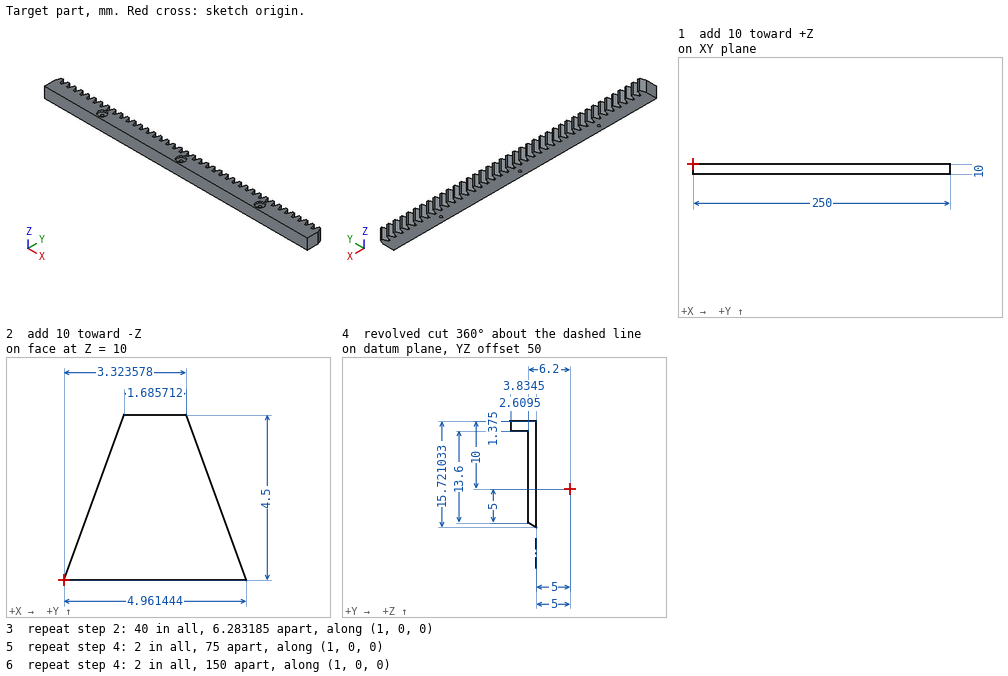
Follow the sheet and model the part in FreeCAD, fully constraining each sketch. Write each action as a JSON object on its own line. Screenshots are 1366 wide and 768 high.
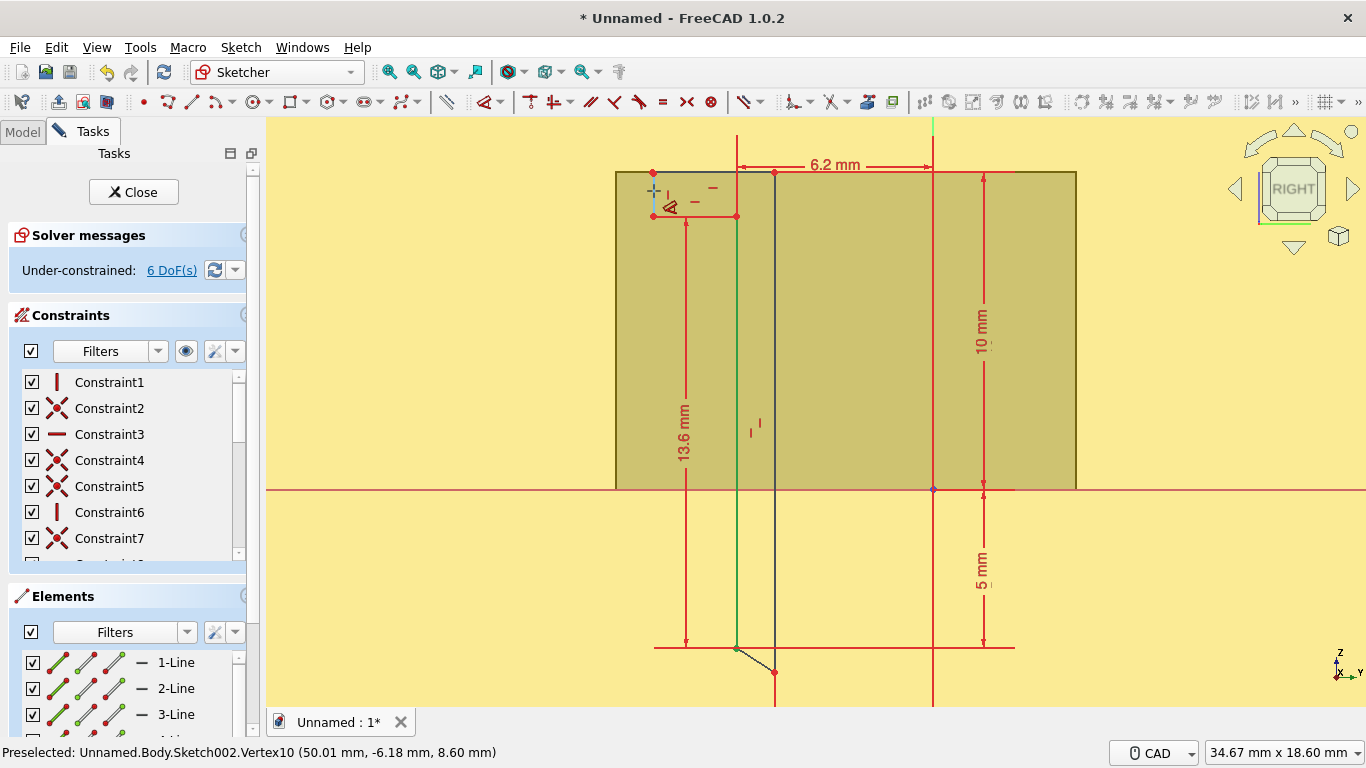
{"action": "left_click", "coordinate": [654, 191]}
{"action": "left_click", "coordinate": [620, 195]}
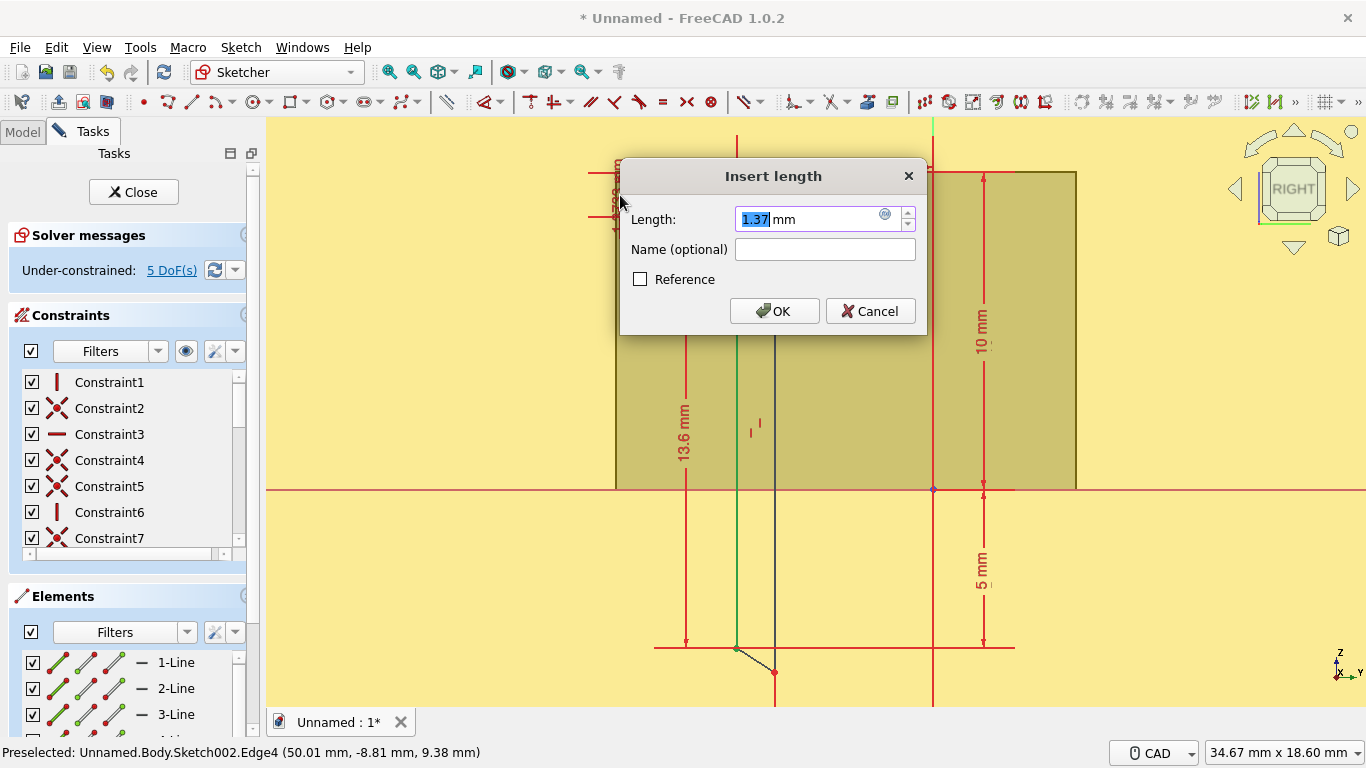
{"action": "type", "text": "1.375"}
{"action": "key", "text": "Return"}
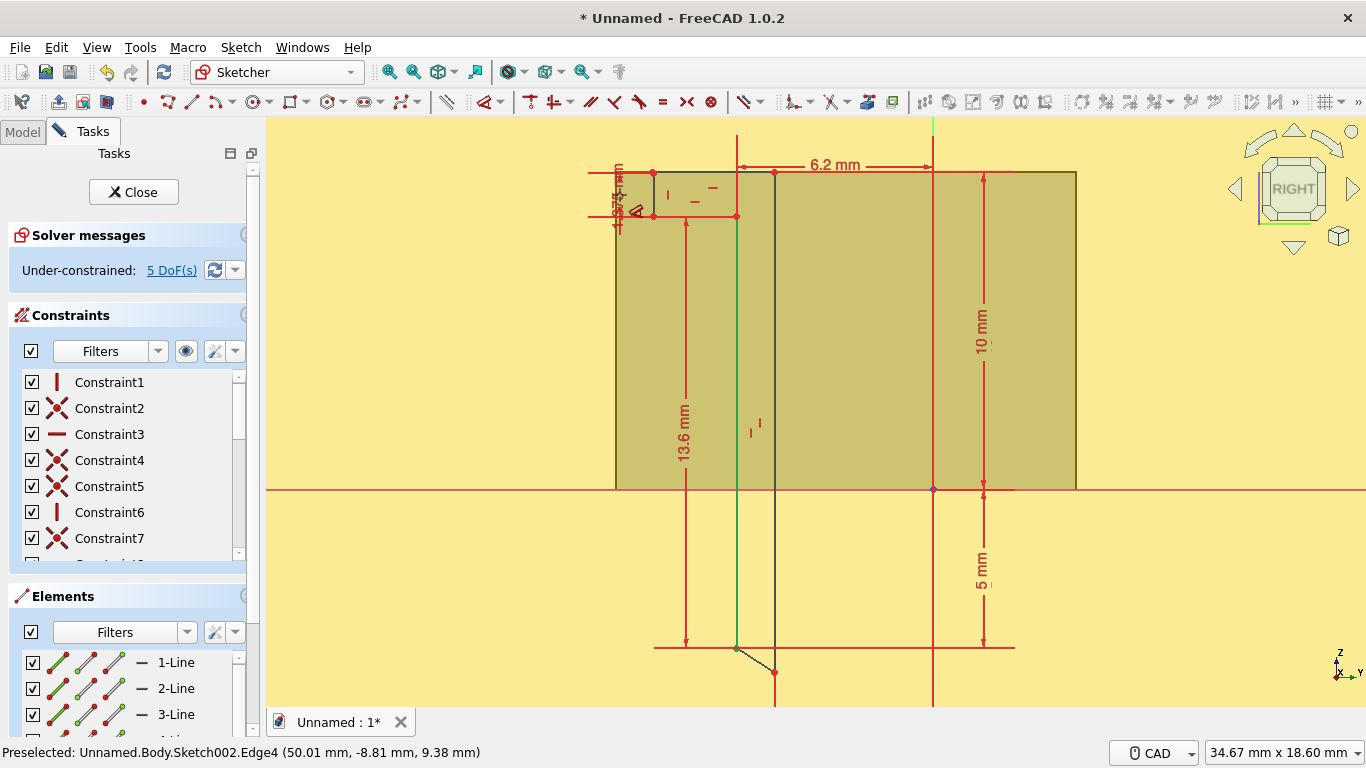
{"action": "left_click", "coordinate": [738, 172]}
{"action": "left_click", "coordinate": [757, 206]}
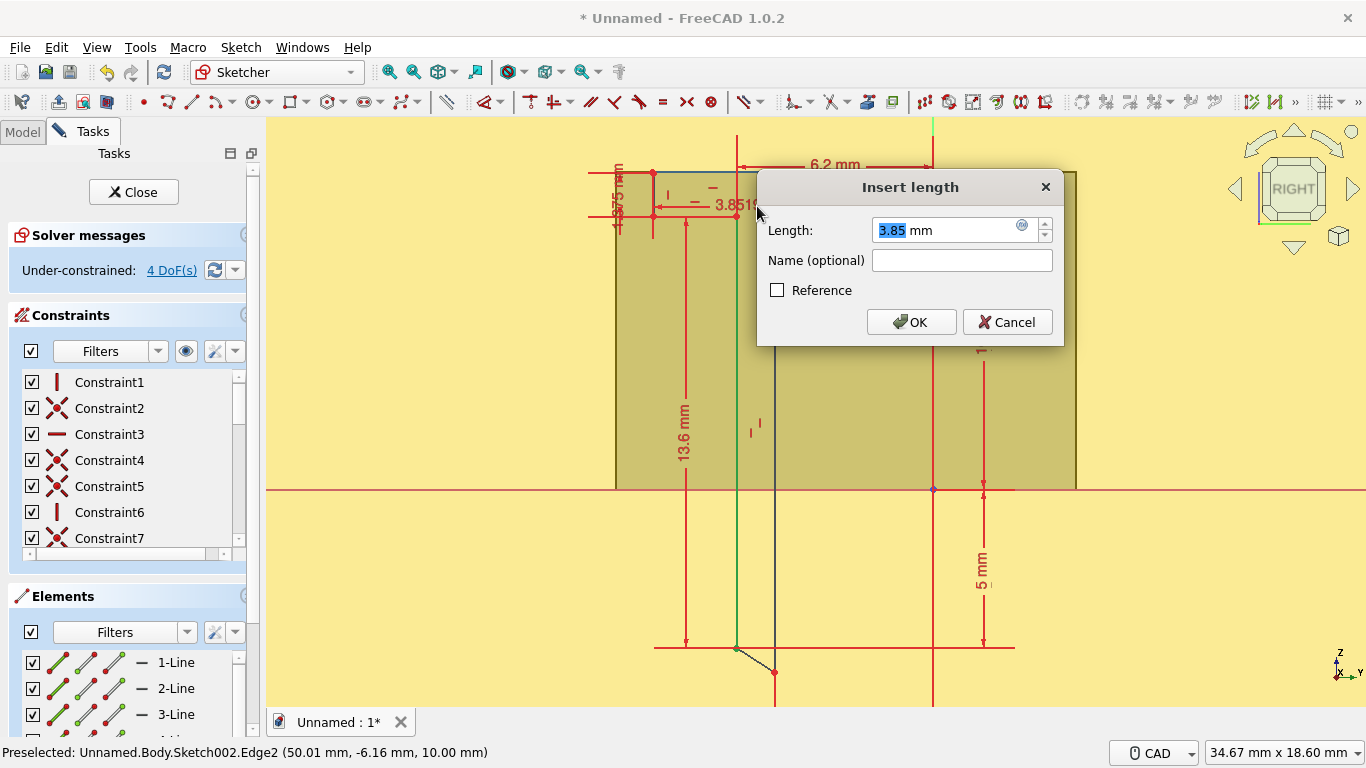
{"action": "type", "text": "3.8345"}
{"action": "key", "text": "Return"}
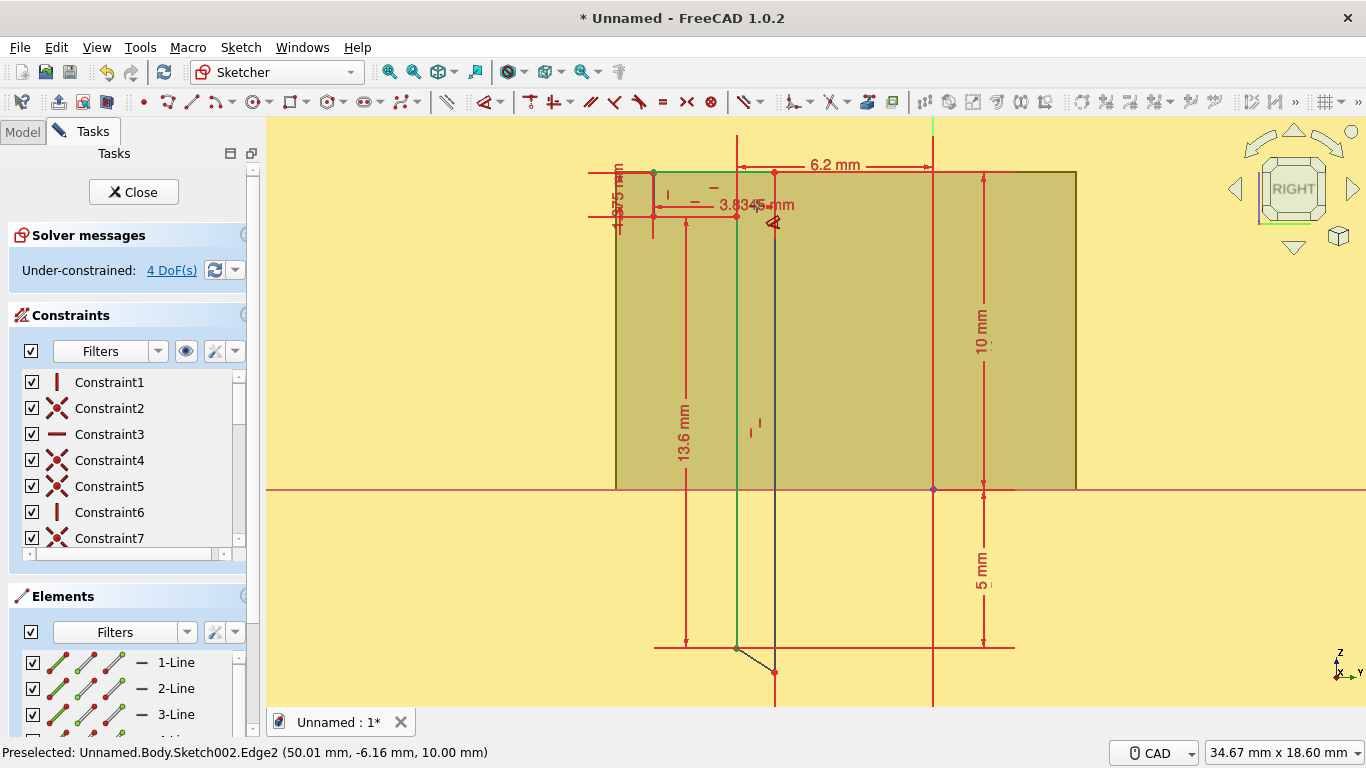
{"action": "left_click", "coordinate": [679, 217]}
{"action": "left_click", "coordinate": [695, 251]}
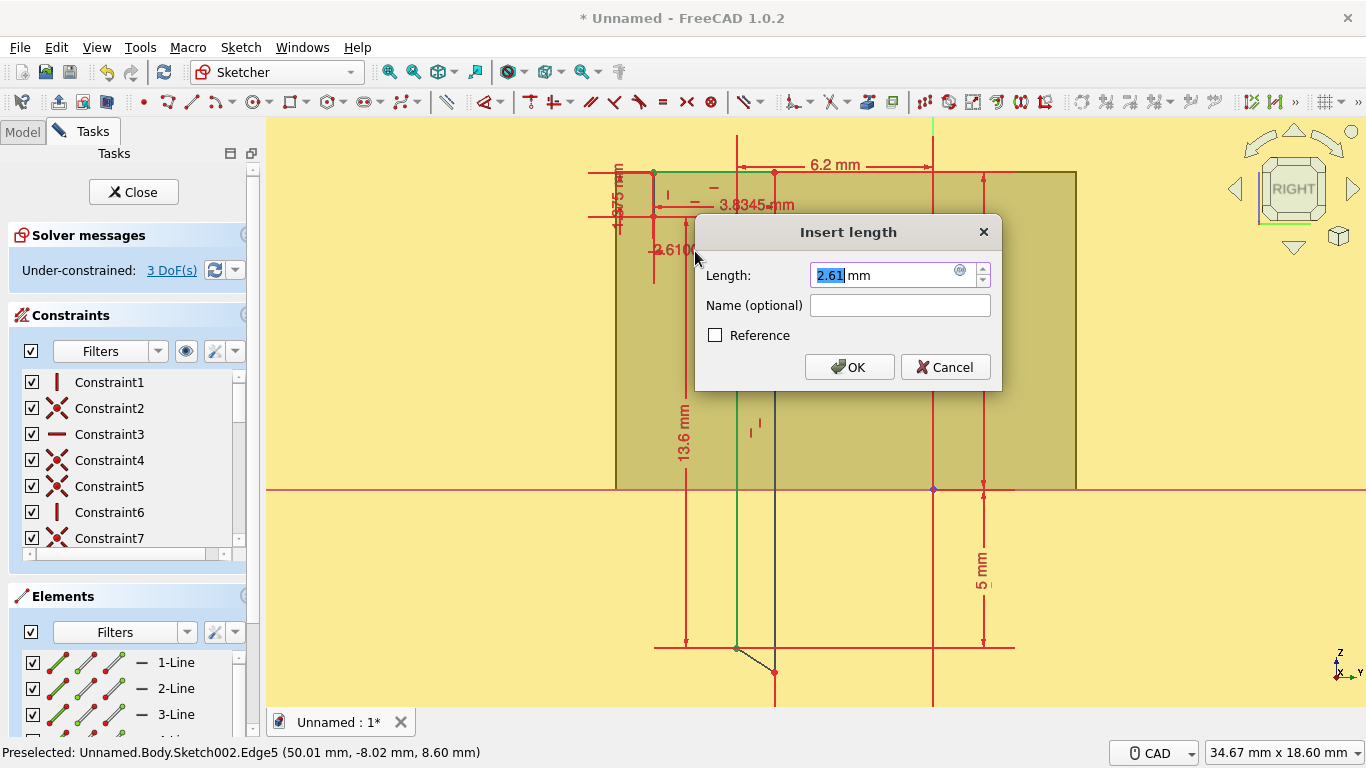
{"action": "type", "text": "2.6095"}
{"action": "key", "text": "Return"}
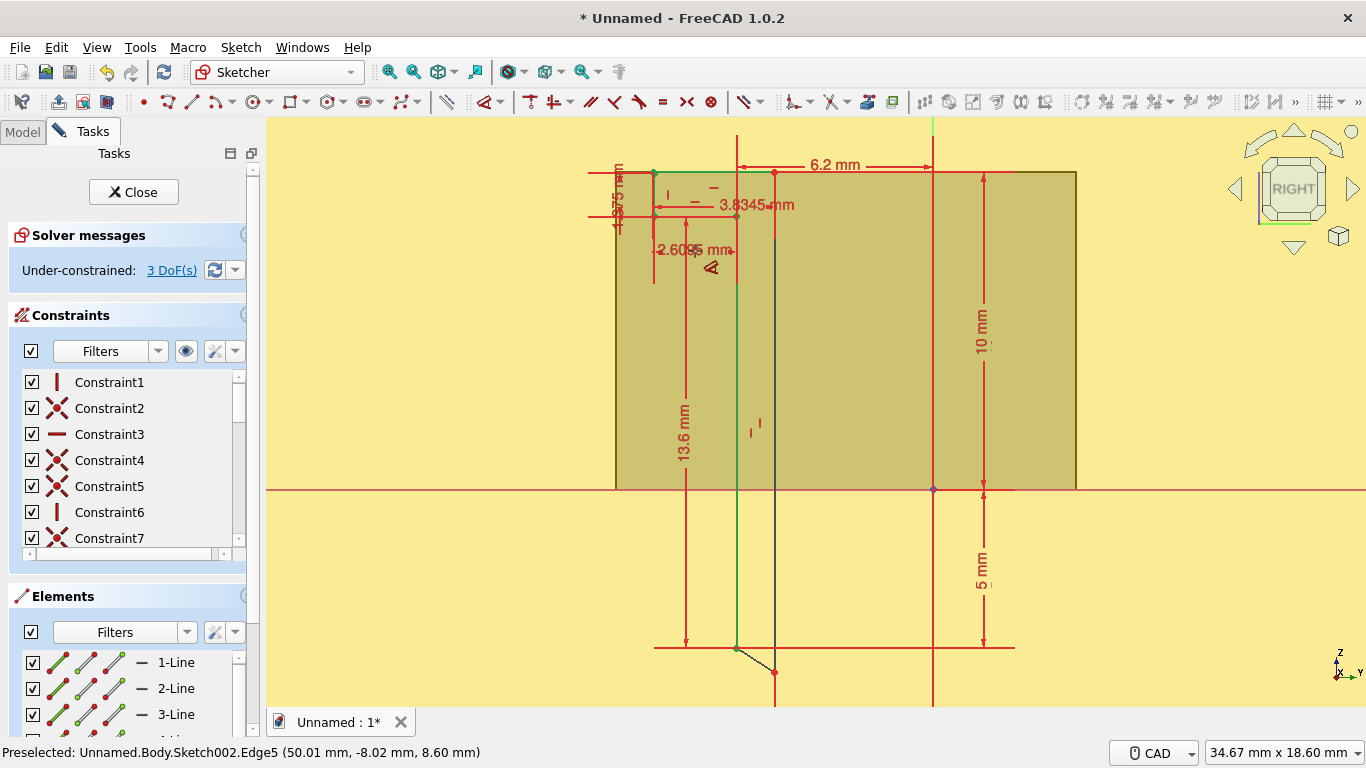
{"action": "left_click", "coordinate": [775, 523]}
{"action": "left_click", "coordinate": [809, 423]}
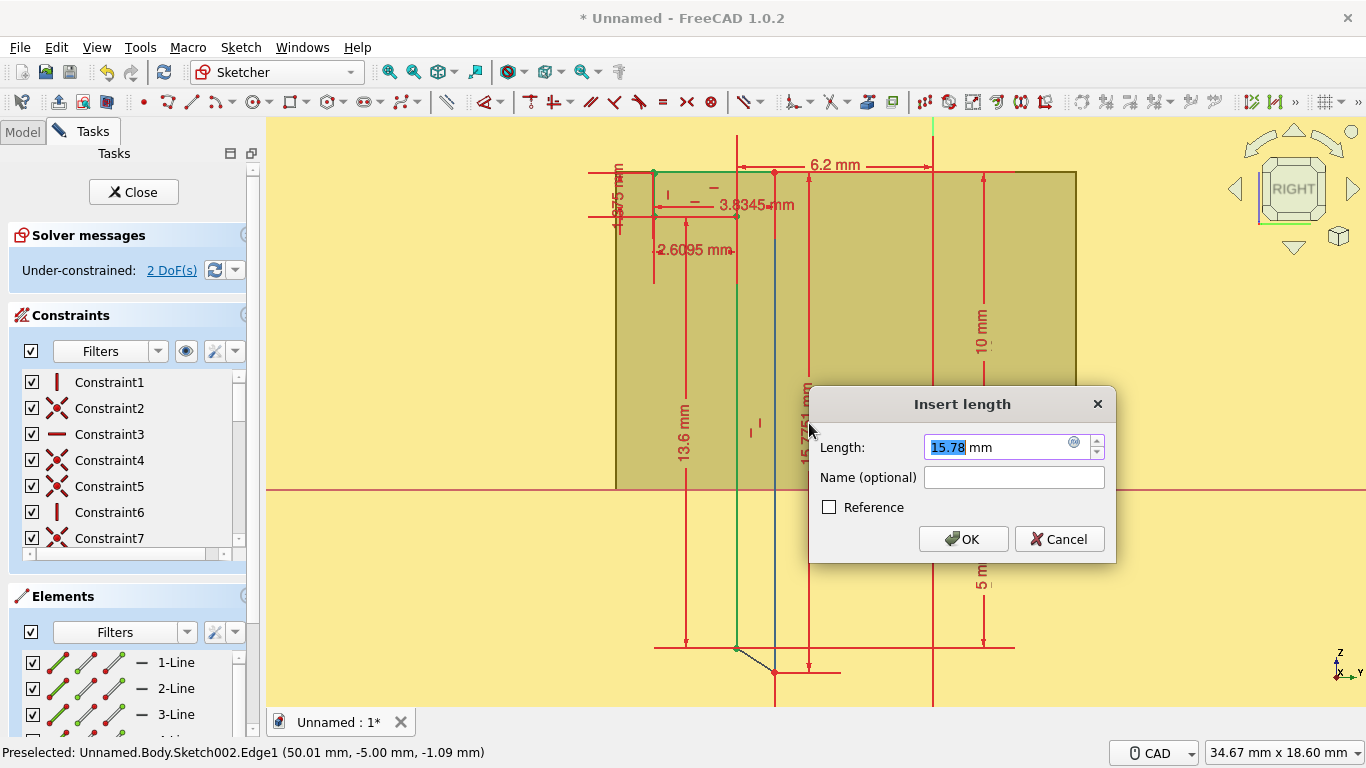
{"action": "type", "text": "15.721033"}
{"action": "key", "text": "Return"}
{"action": "key", "text": "Escape"}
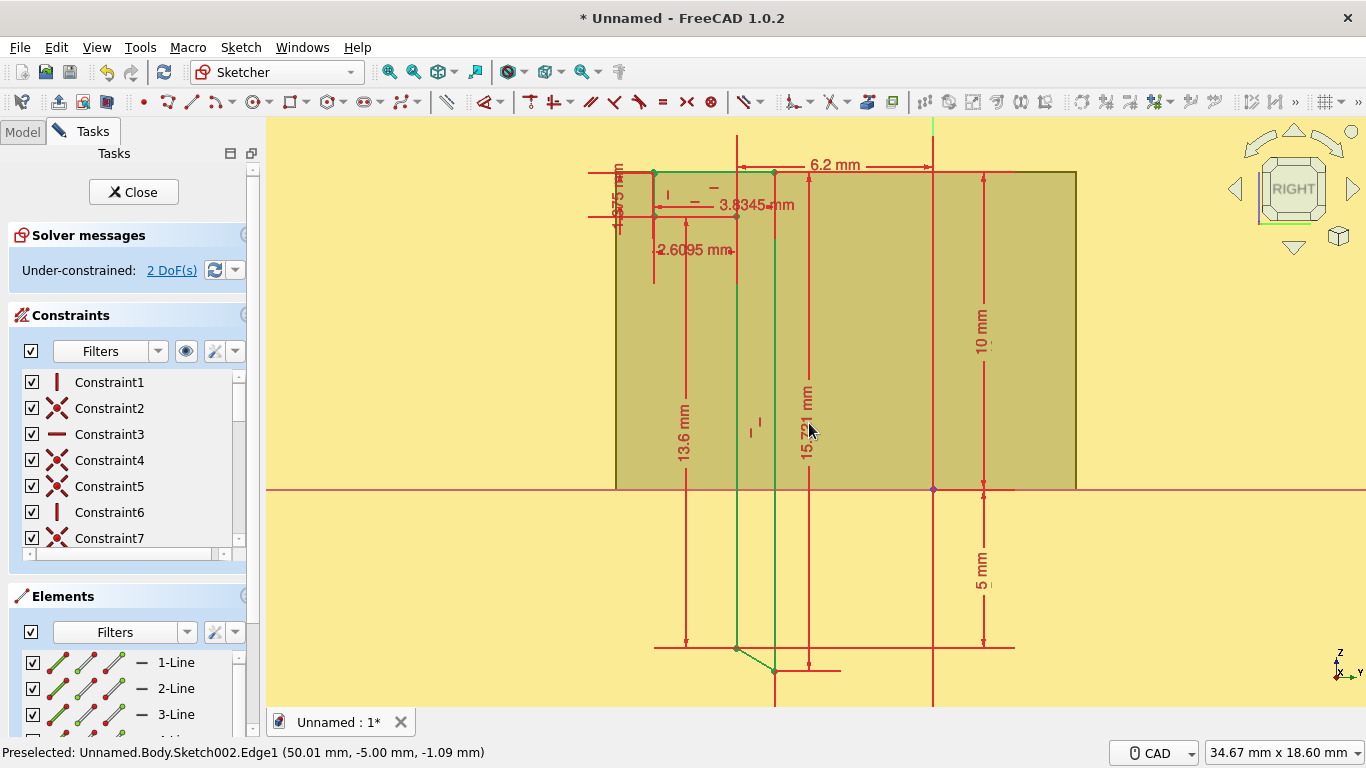
{"action": "left_click", "coordinate": [134, 192]}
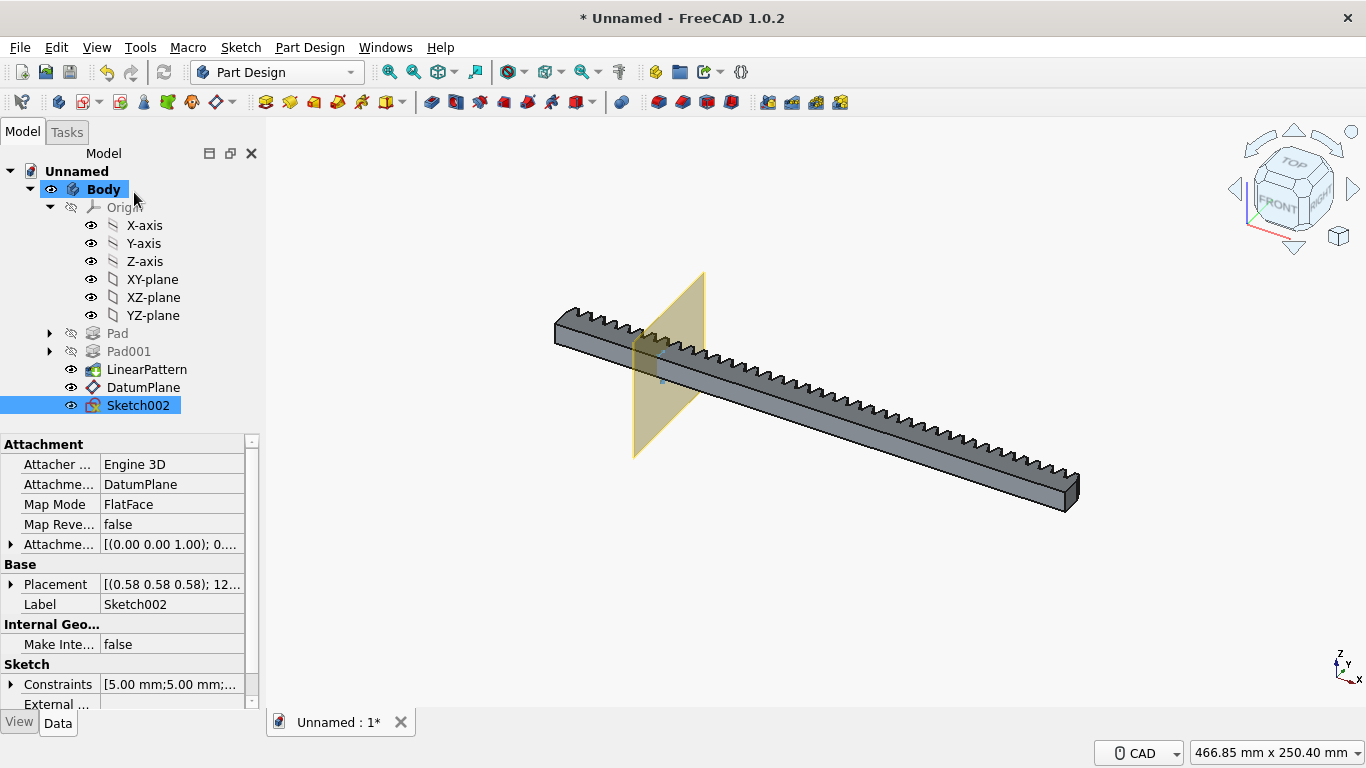
{"action": "left_click", "coordinate": [480, 102]}